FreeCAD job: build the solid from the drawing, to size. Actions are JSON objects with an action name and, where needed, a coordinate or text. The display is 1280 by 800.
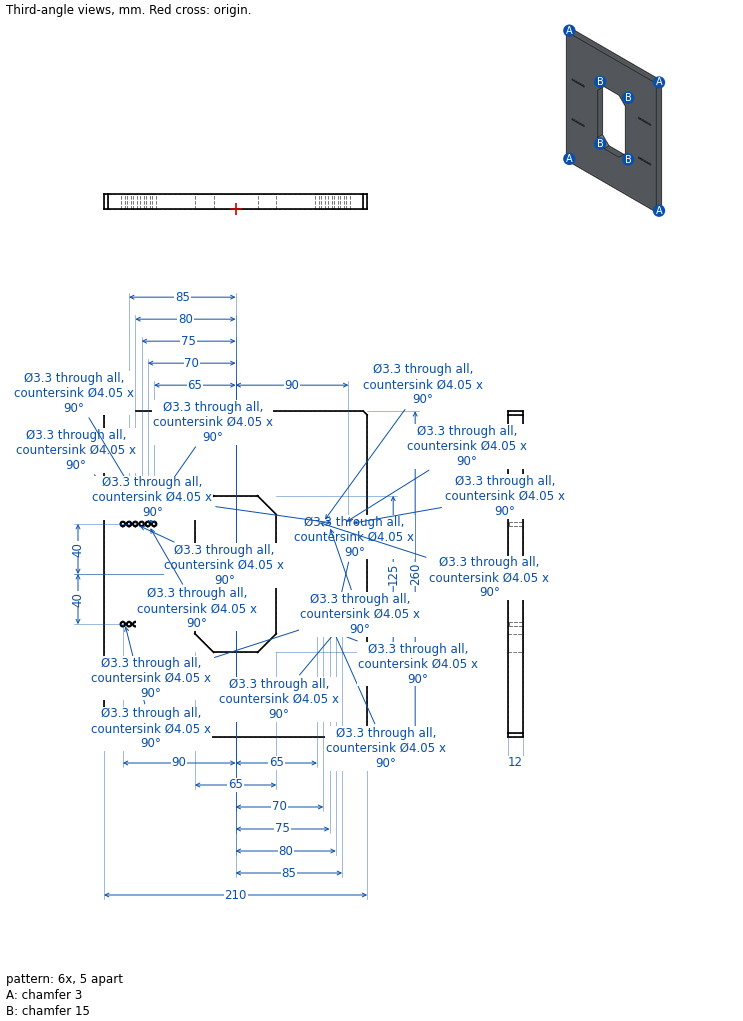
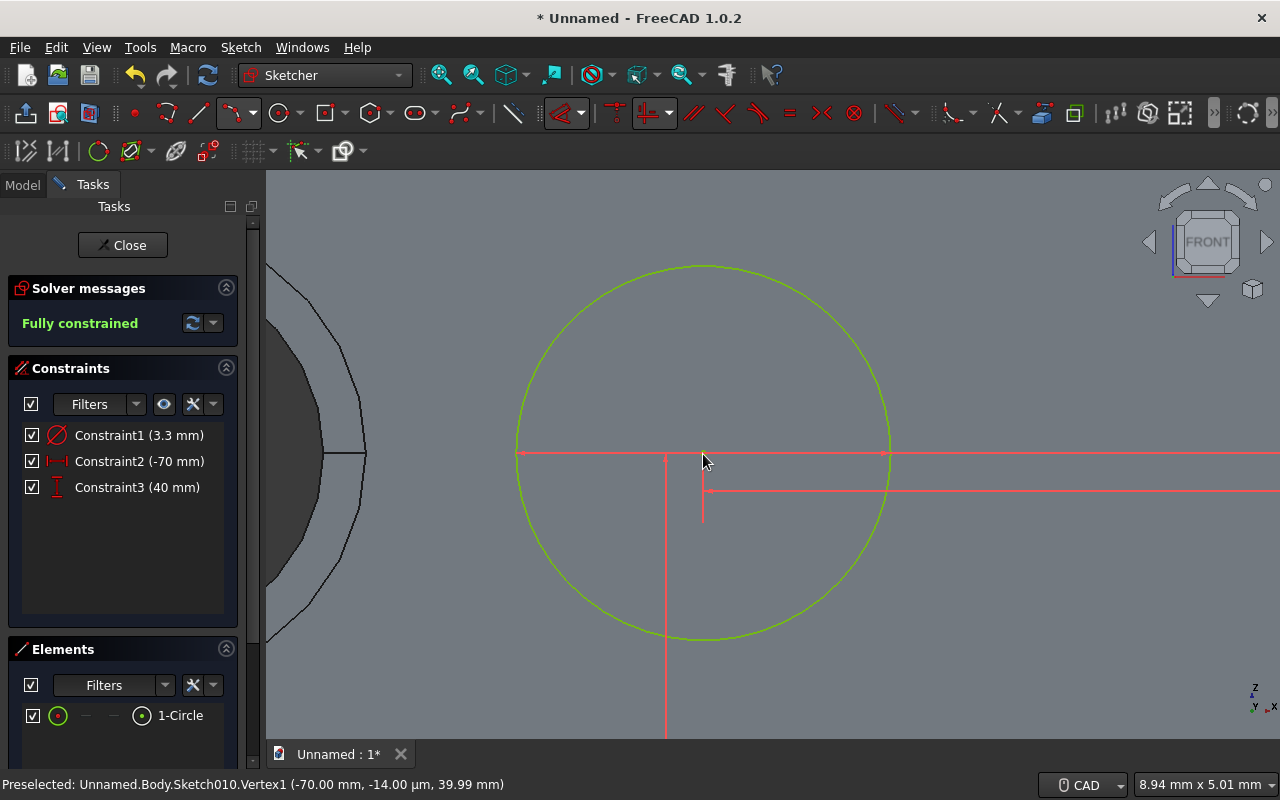
{"action": "left_click", "coordinate": [123, 245]}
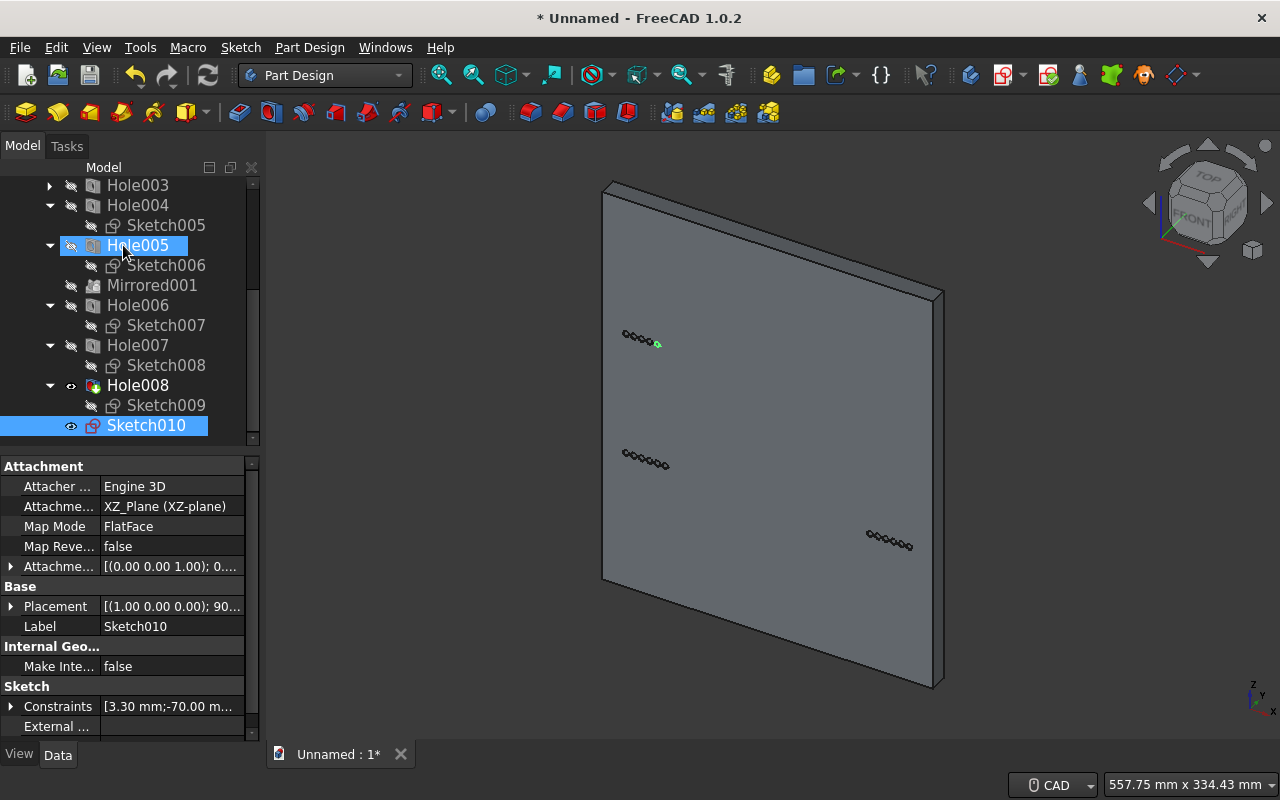
{"action": "left_click", "coordinate": [272, 112]}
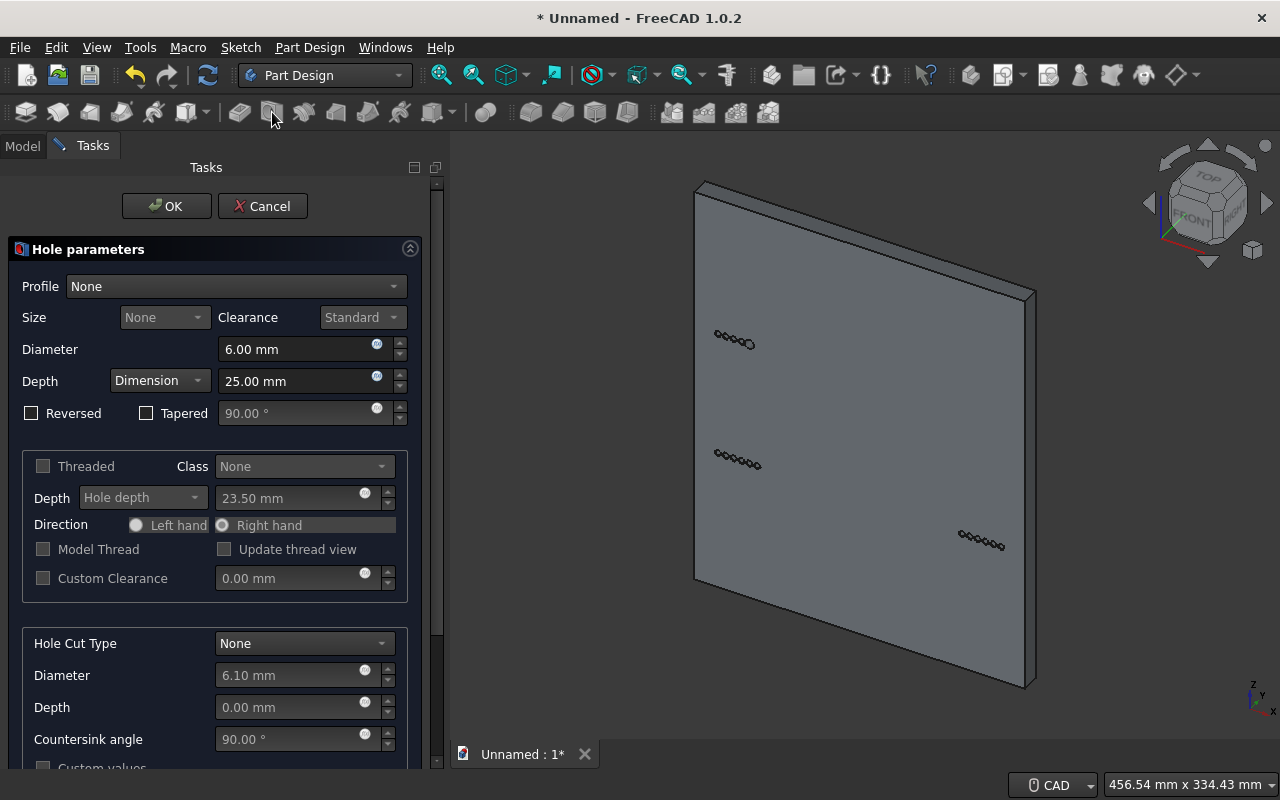
{"action": "triple_click", "coordinate": [305, 349]}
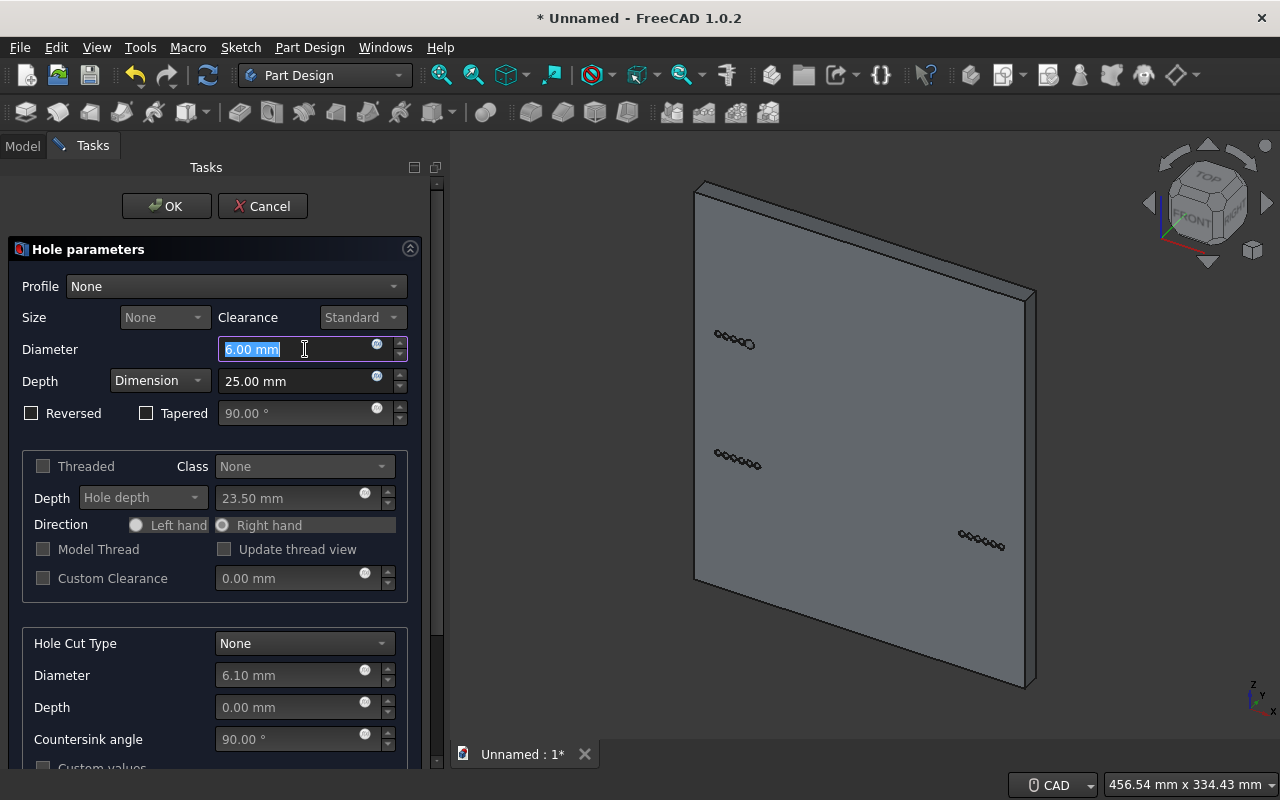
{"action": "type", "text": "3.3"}
{"action": "key", "text": "Tab"}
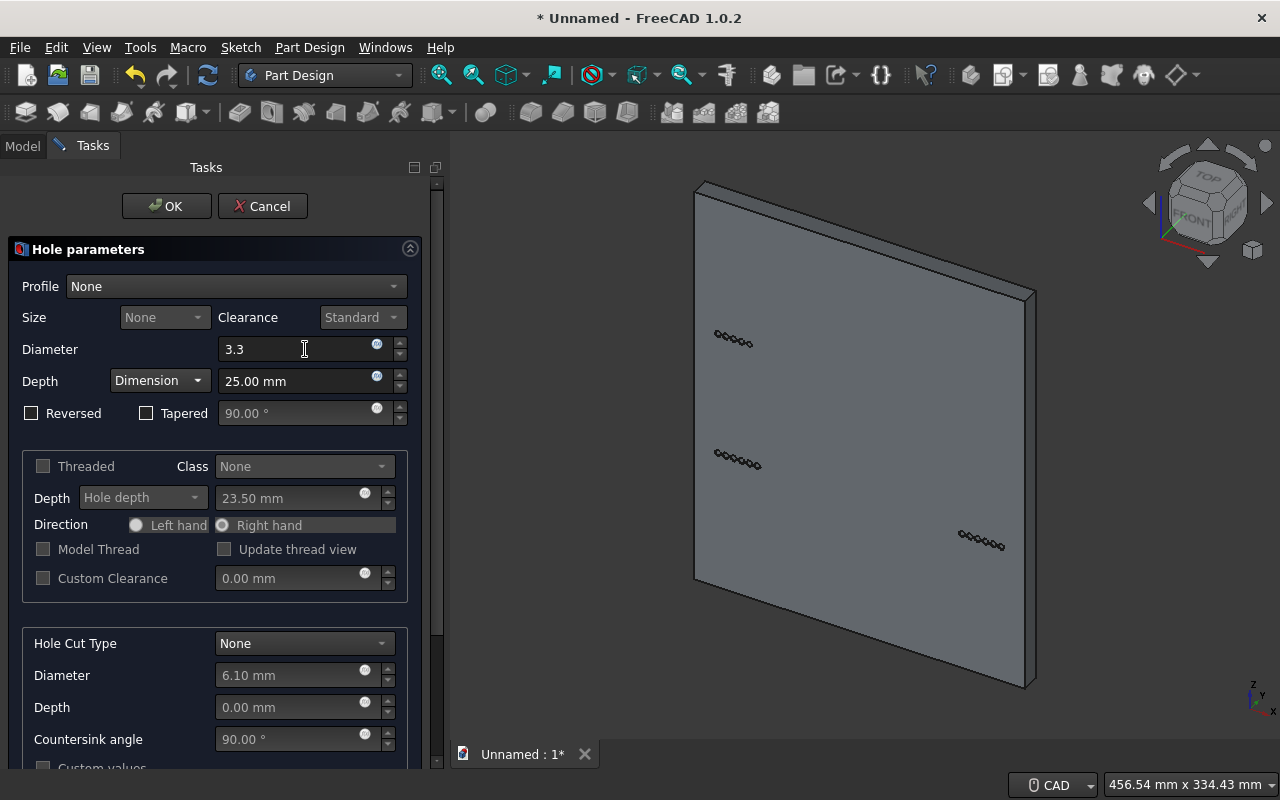
{"action": "left_click", "coordinate": [161, 380]}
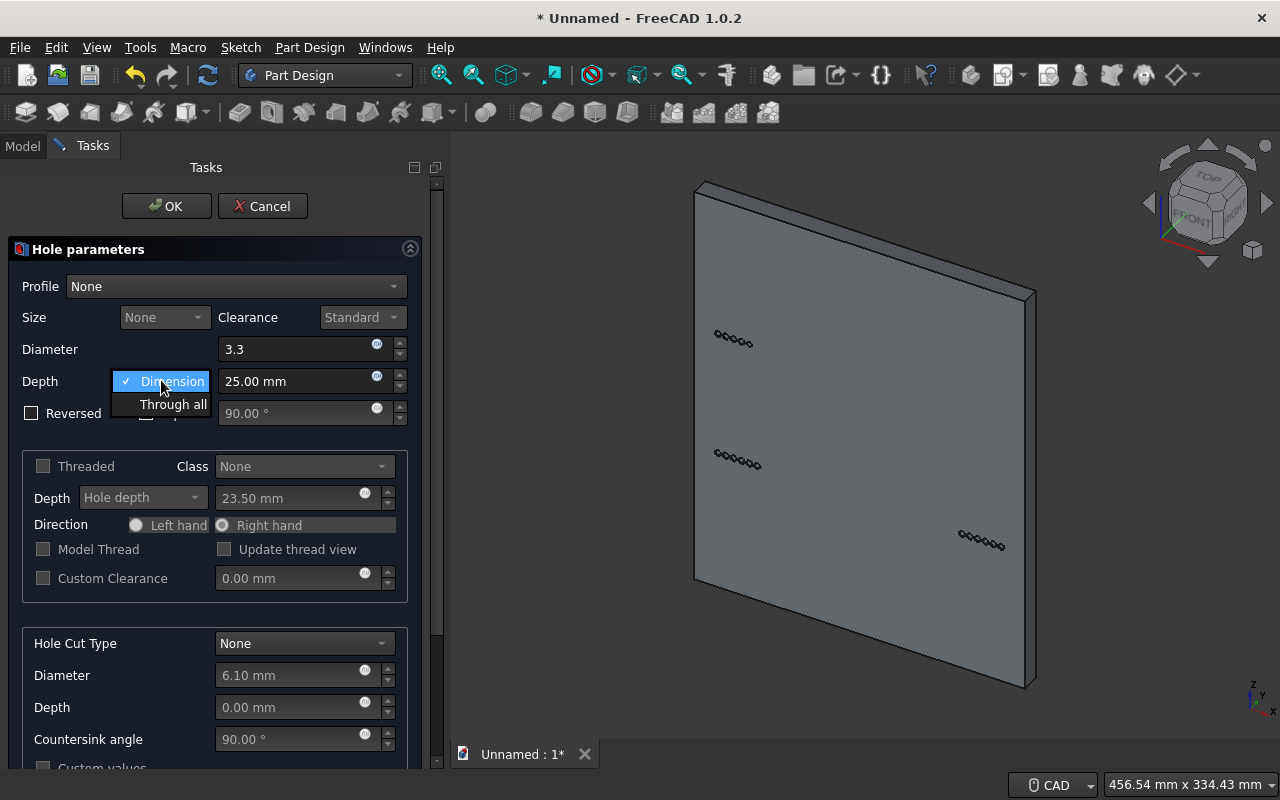
{"action": "left_click", "coordinate": [160, 404]}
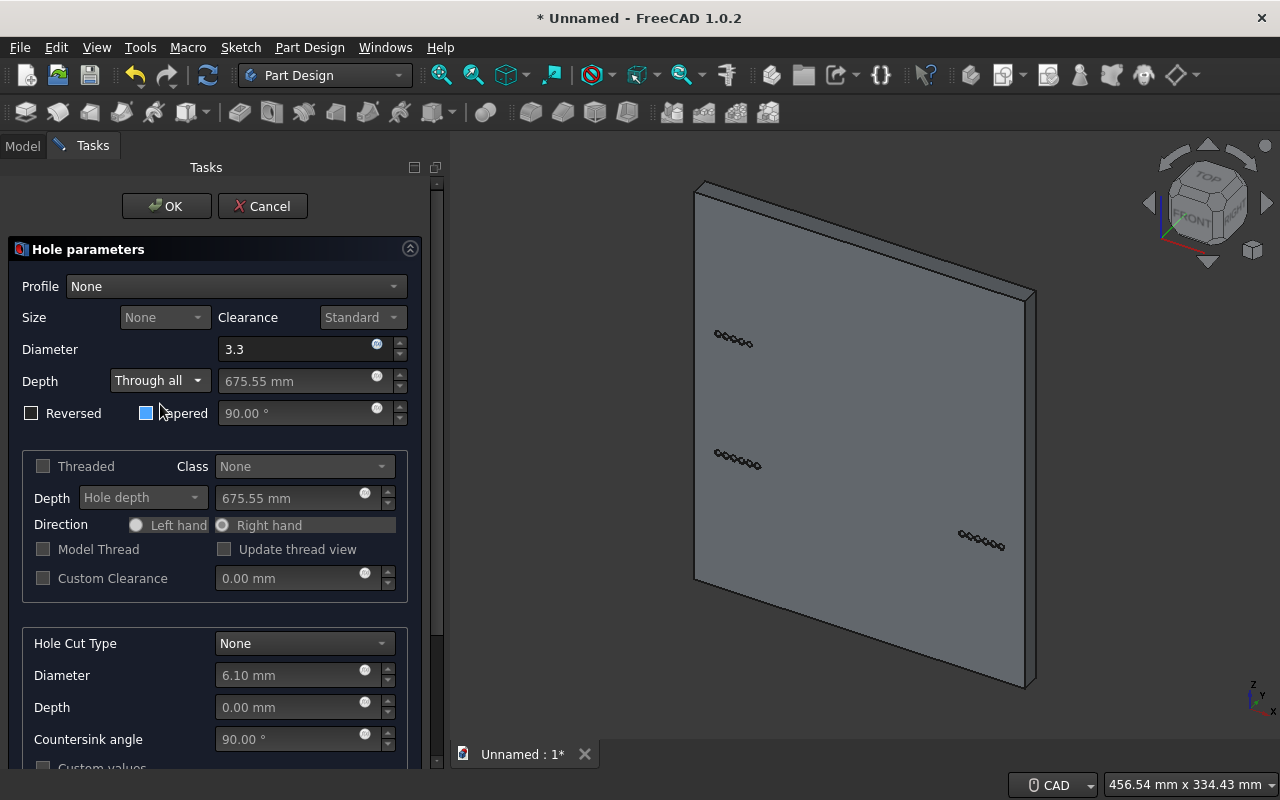
{"action": "left_click", "coordinate": [306, 644]}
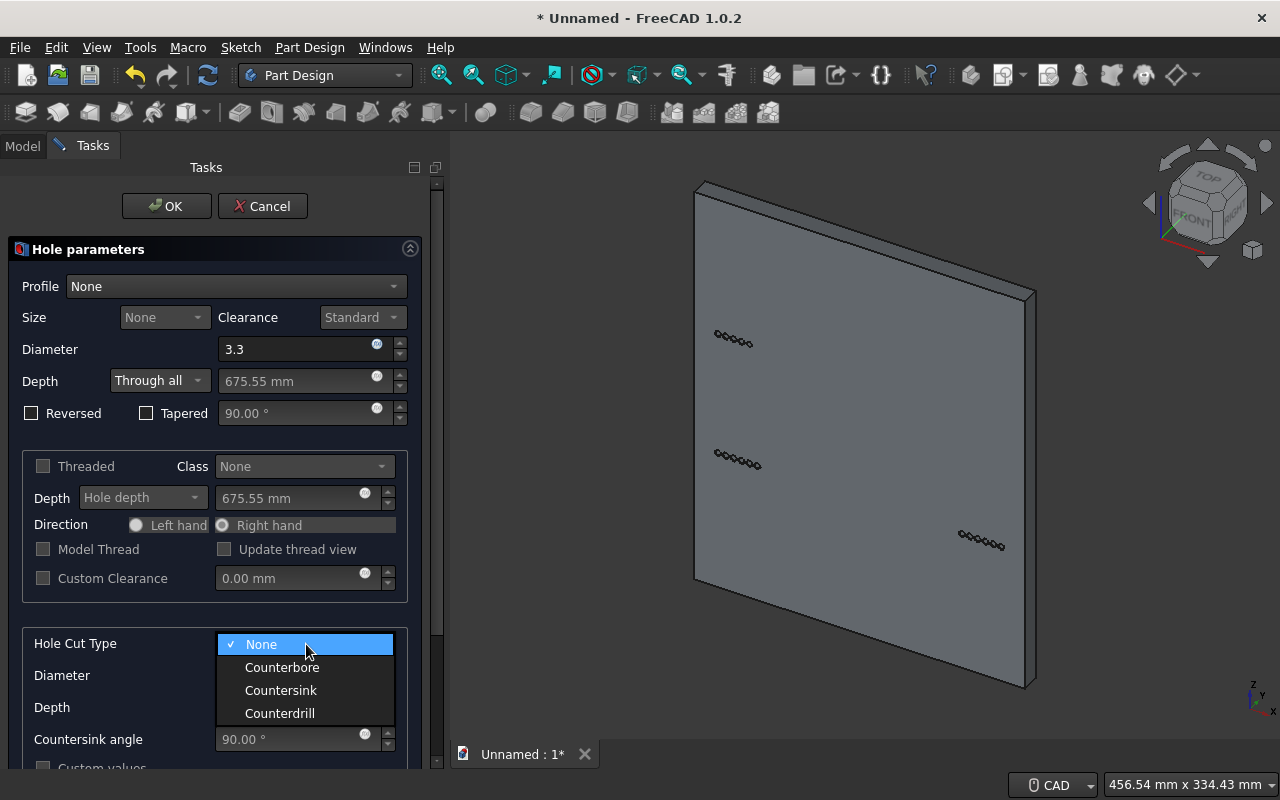
{"action": "left_click", "coordinate": [304, 690]}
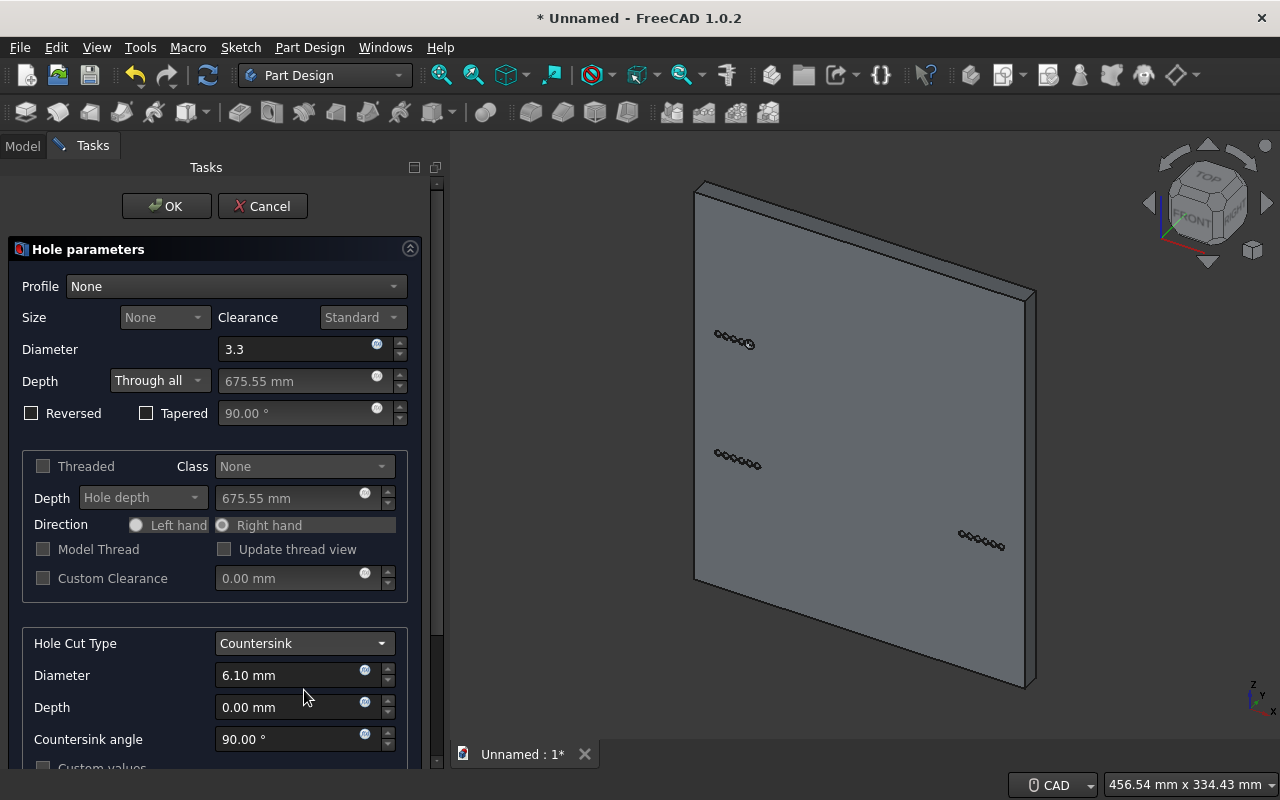
{"action": "triple_click", "coordinate": [298, 675]}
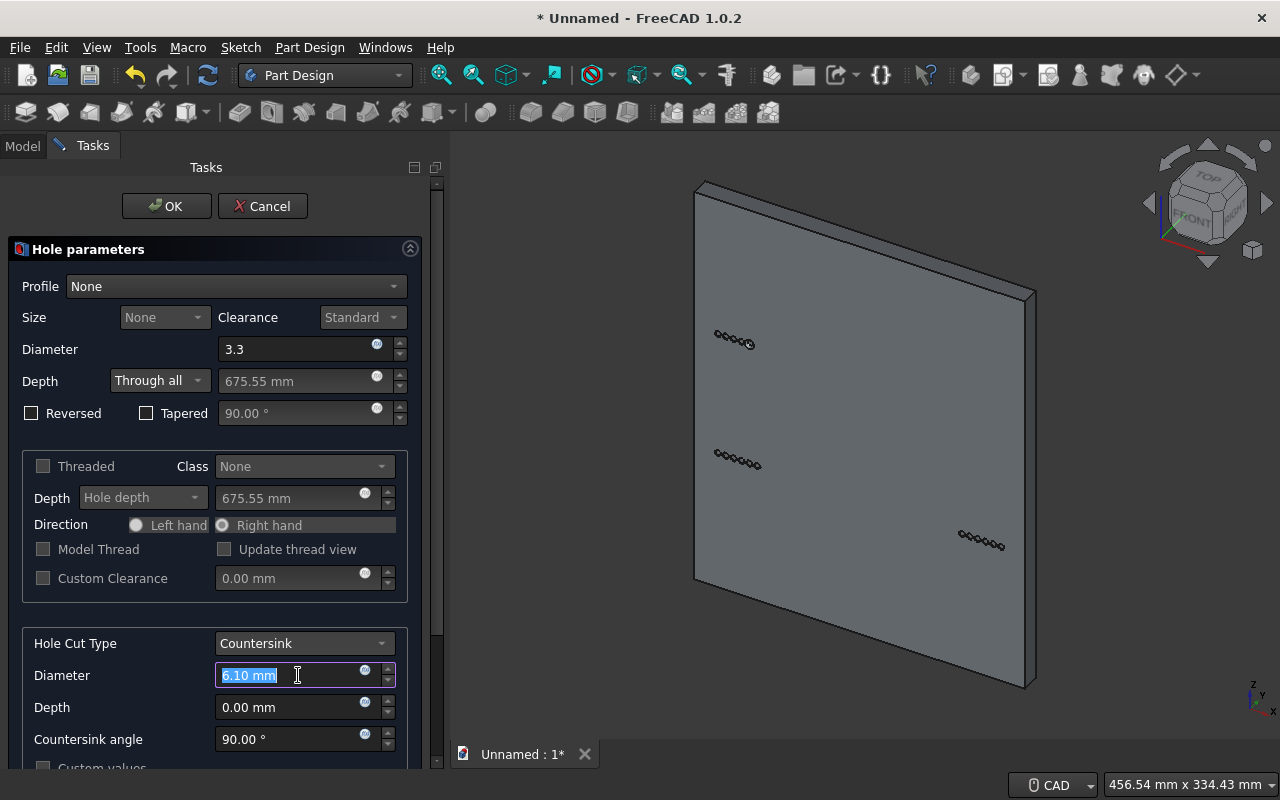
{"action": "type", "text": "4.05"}
{"action": "key", "text": "Tab"}